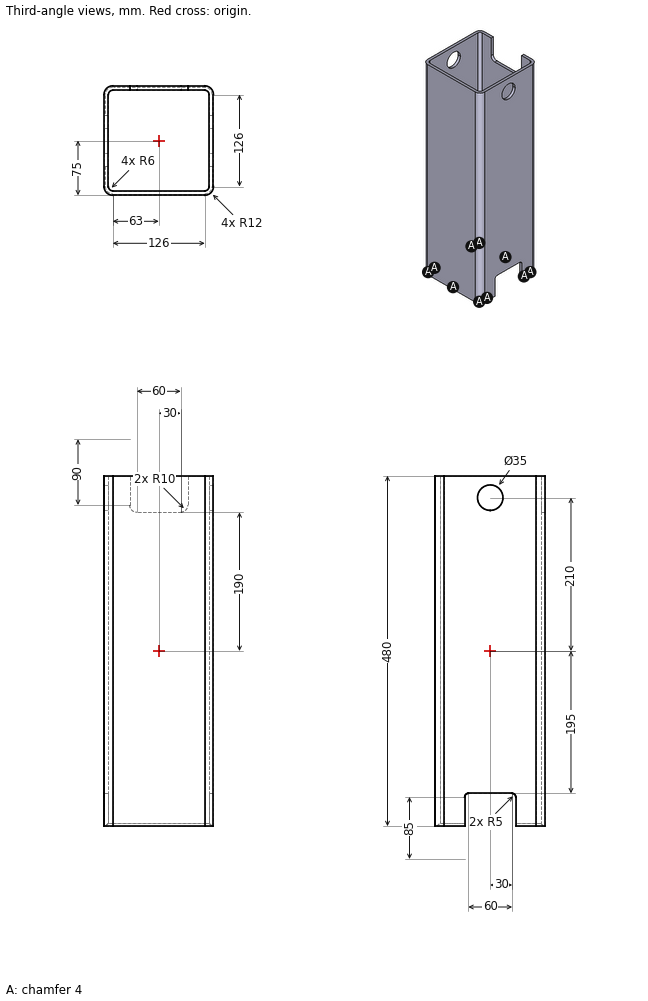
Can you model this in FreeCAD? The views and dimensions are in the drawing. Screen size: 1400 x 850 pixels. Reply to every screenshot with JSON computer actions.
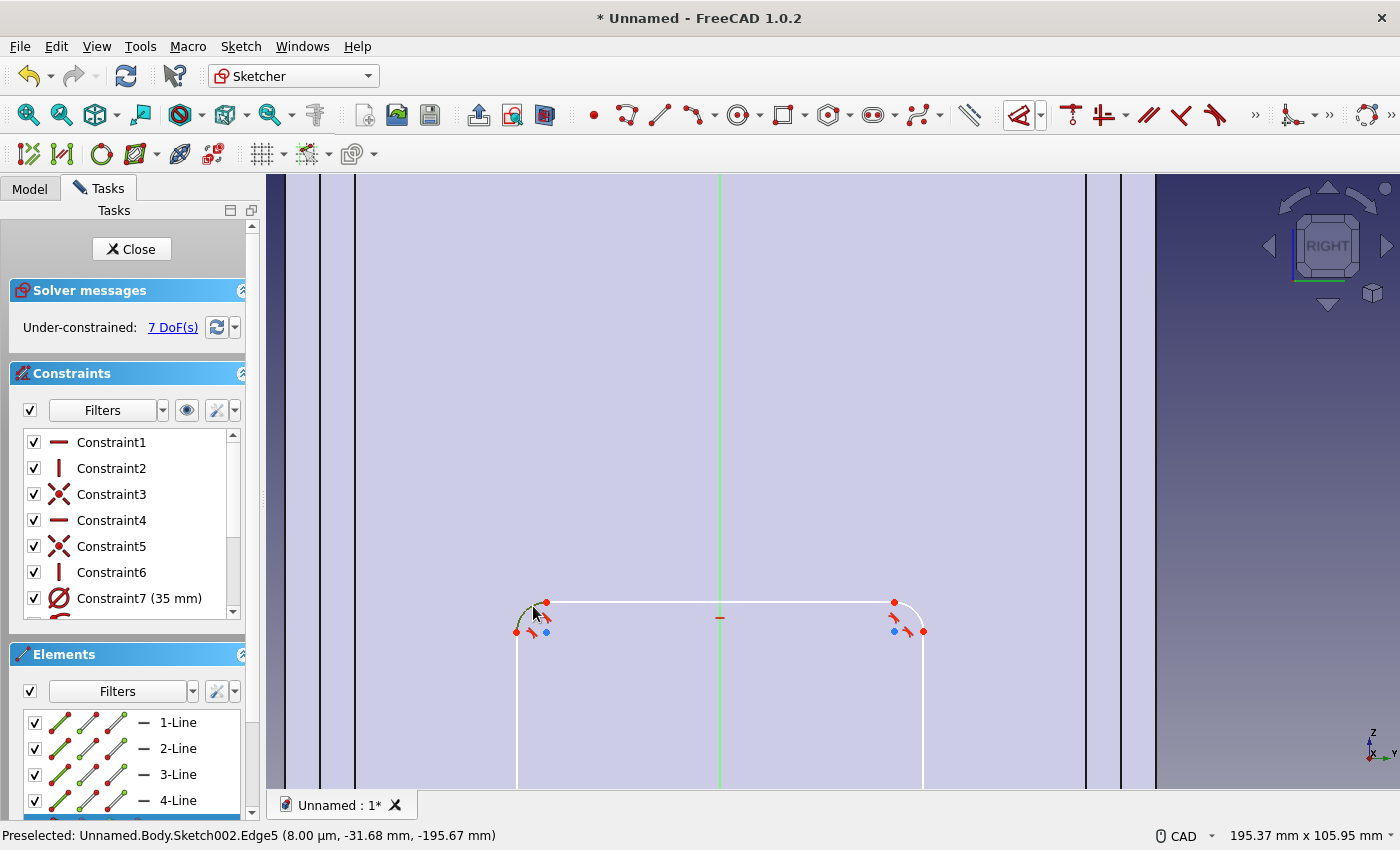
{"action": "left_click", "coordinate": [920, 619]}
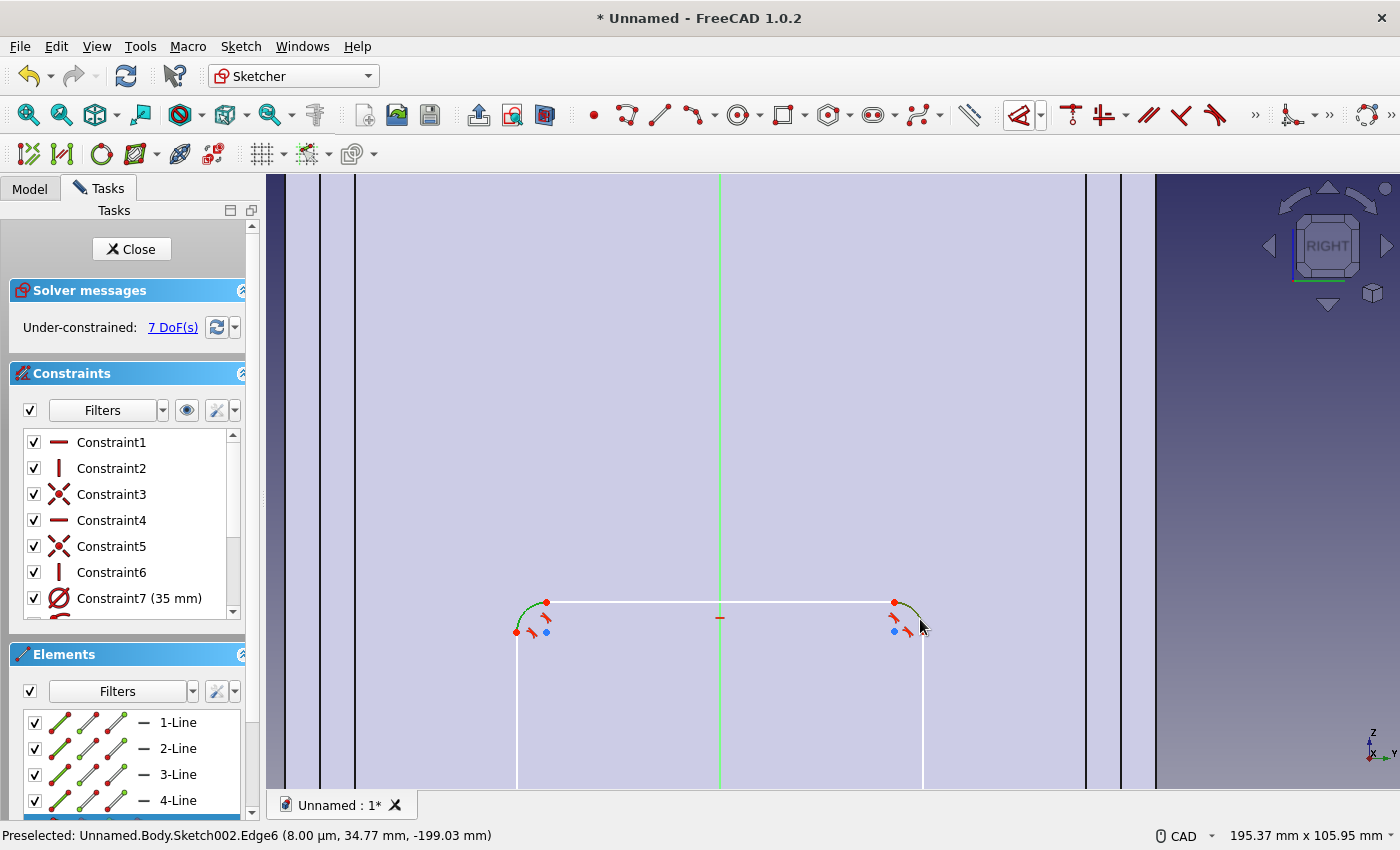
{"action": "key", "text": "e"}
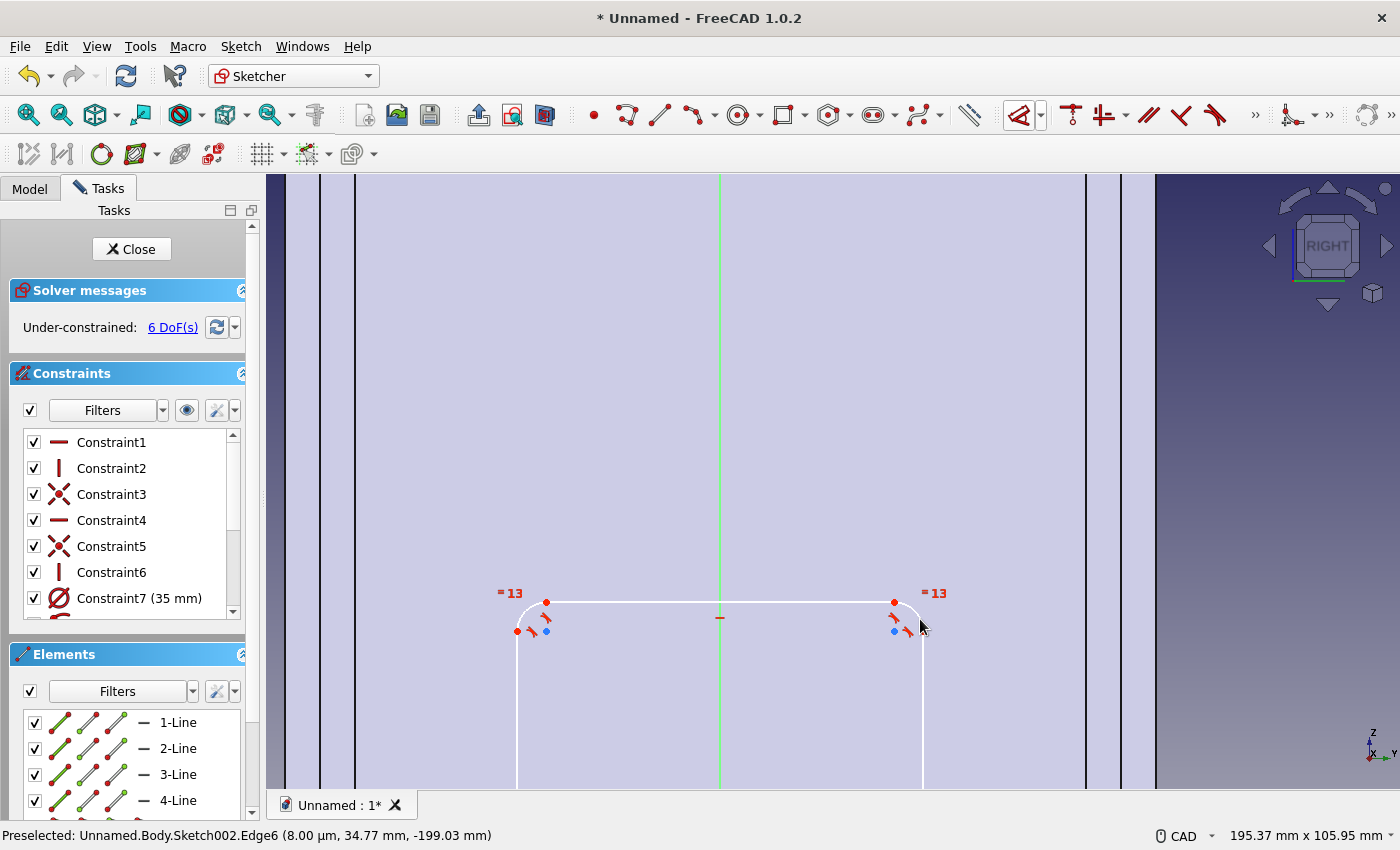
{"action": "scroll", "coordinate": [533, 606], "scroll_direction": "up", "scroll_amount": 2}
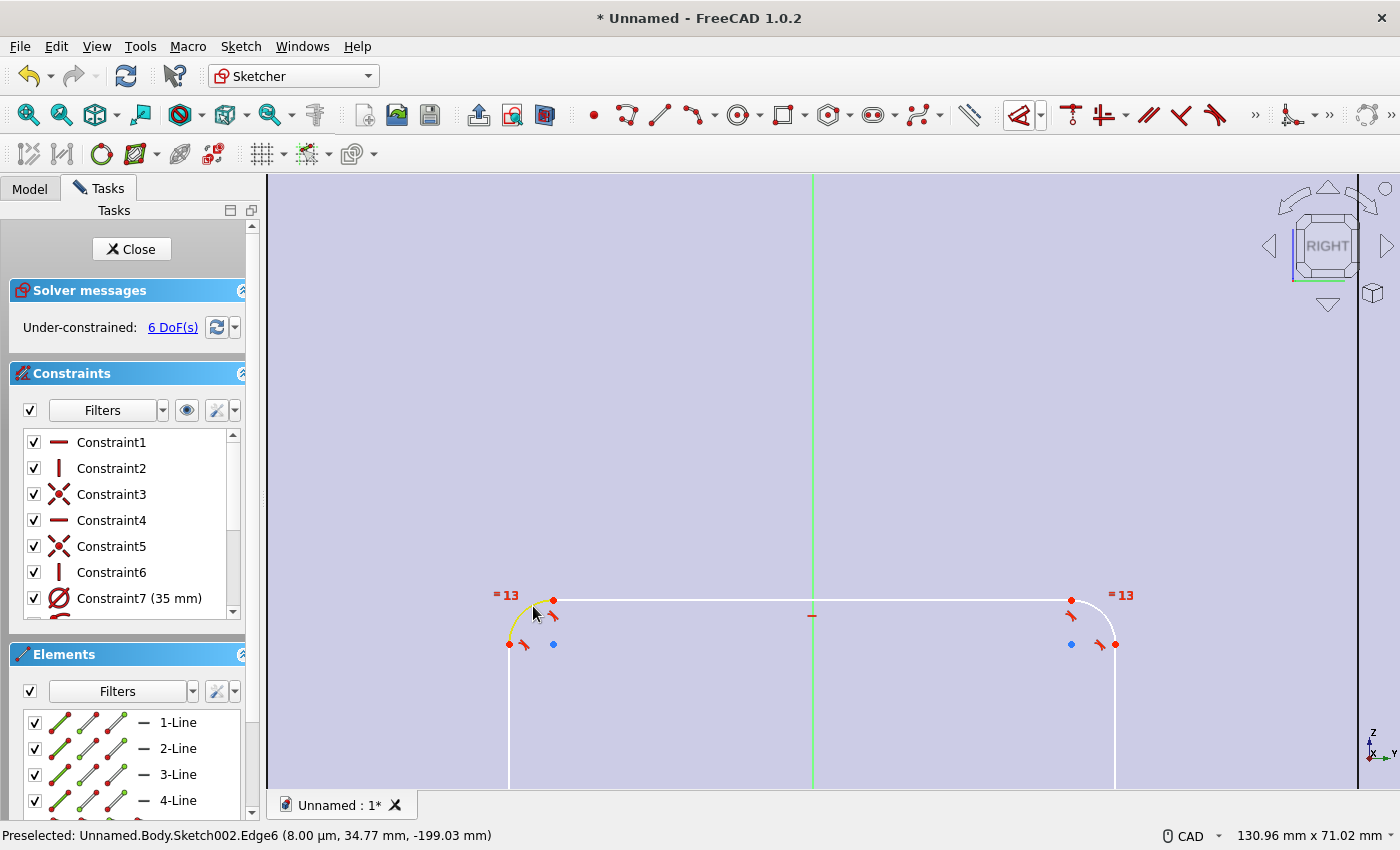
{"action": "left_click", "coordinate": [533, 605]}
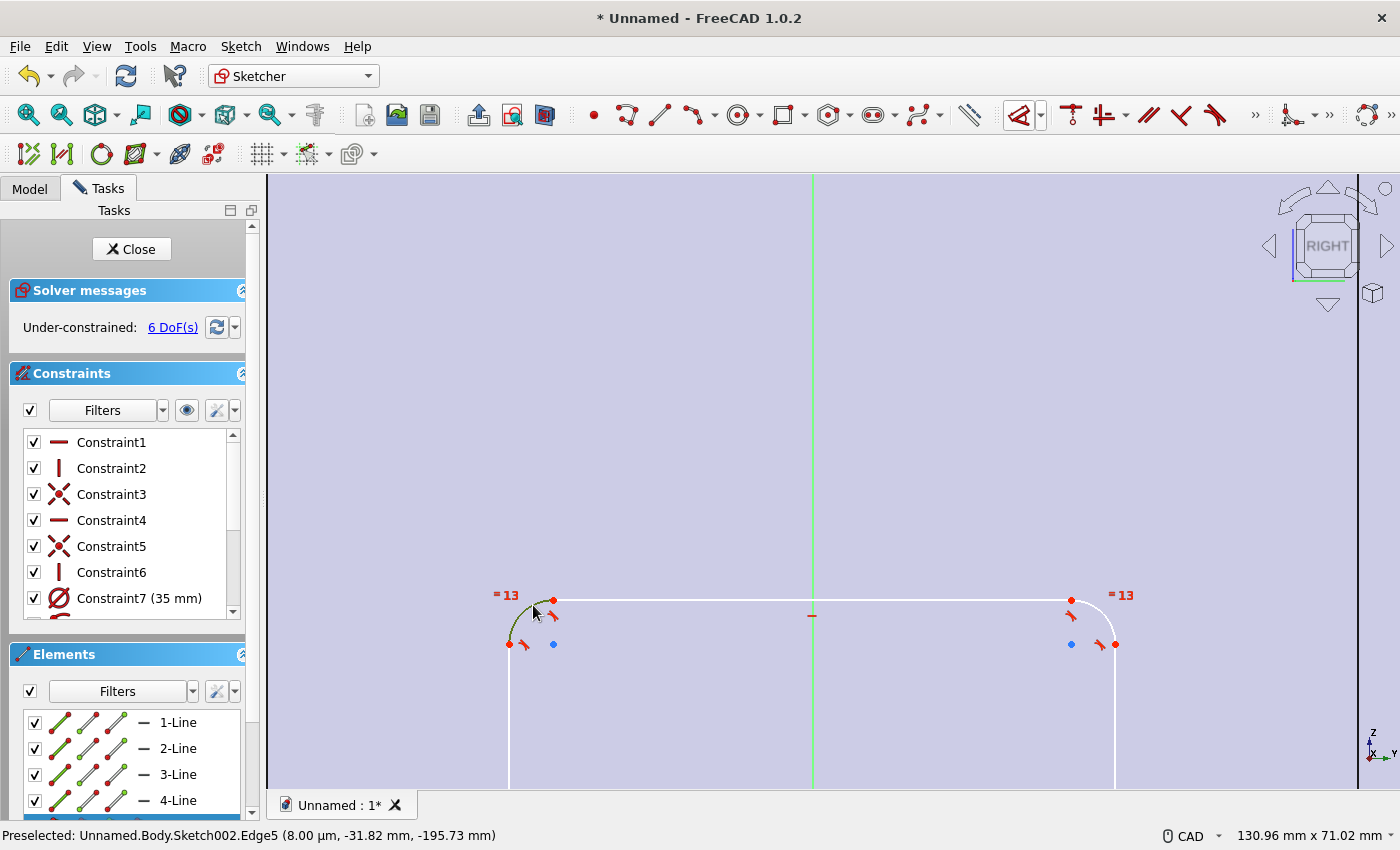
{"action": "left_click", "coordinate": [1040, 116]}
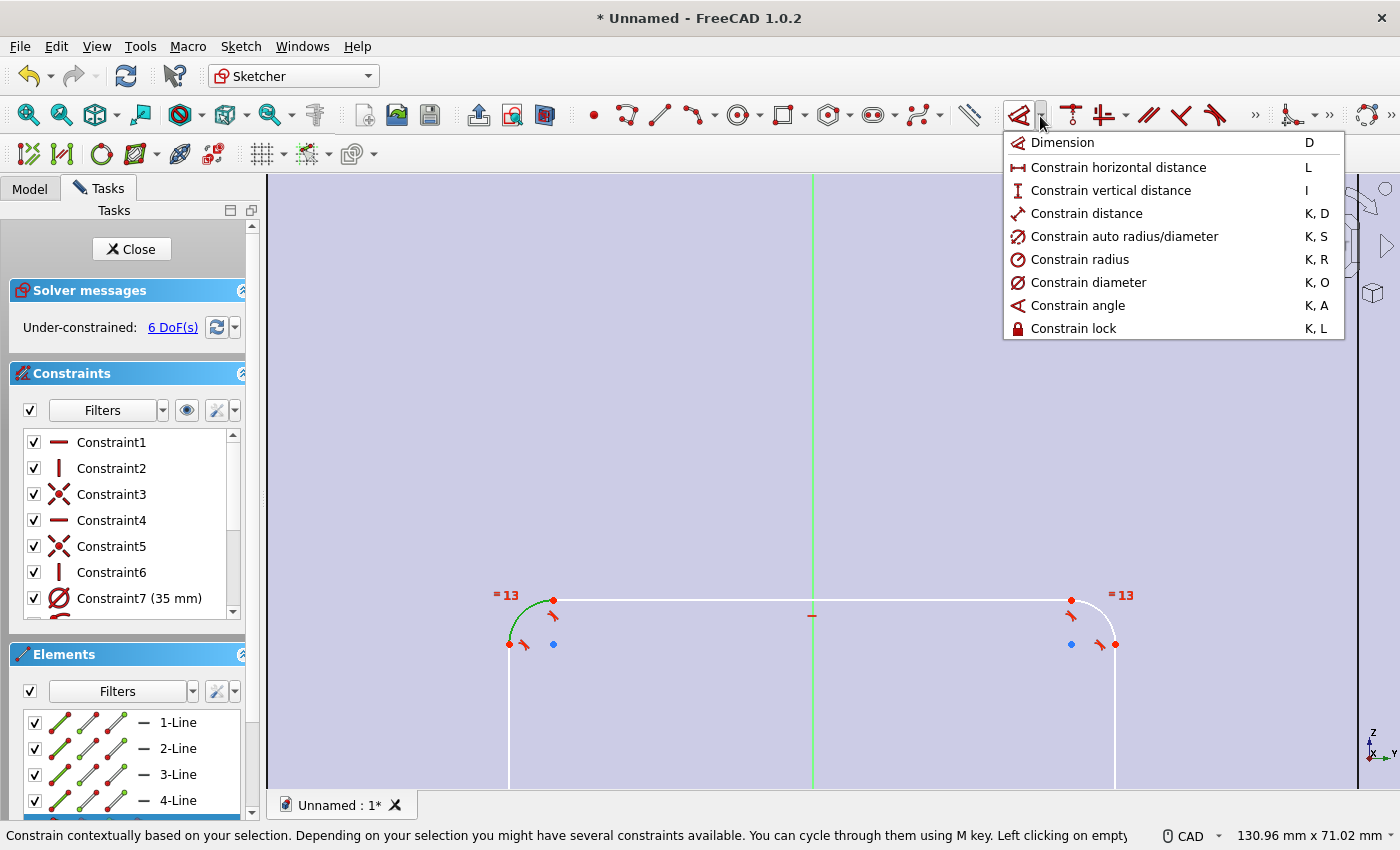
{"action": "left_click", "coordinate": [1174, 260]}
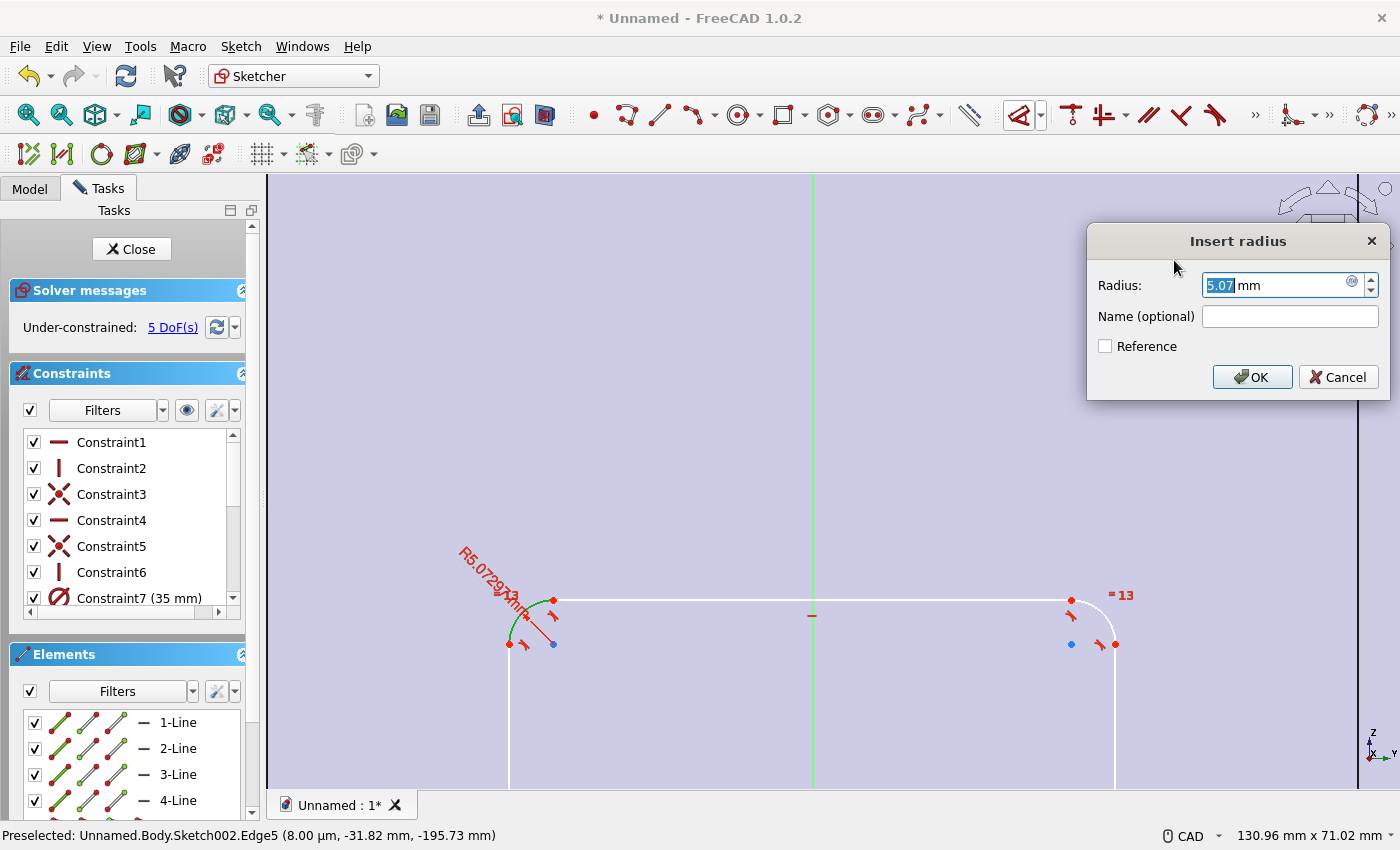
{"action": "type", "text": "5"}
{"action": "key", "text": "Return"}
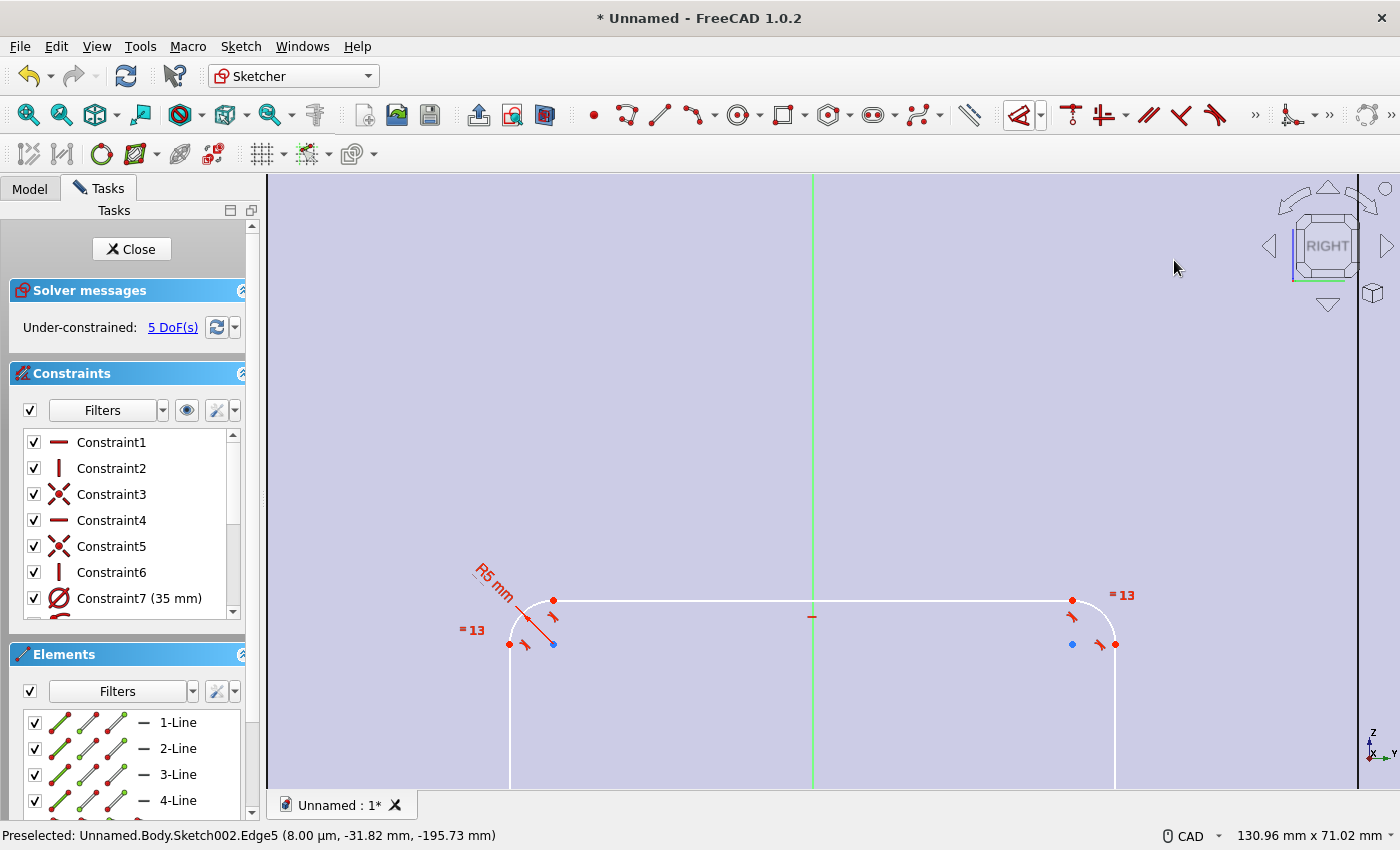
{"action": "scroll", "coordinate": [760, 614], "scroll_direction": "down", "scroll_amount": 12}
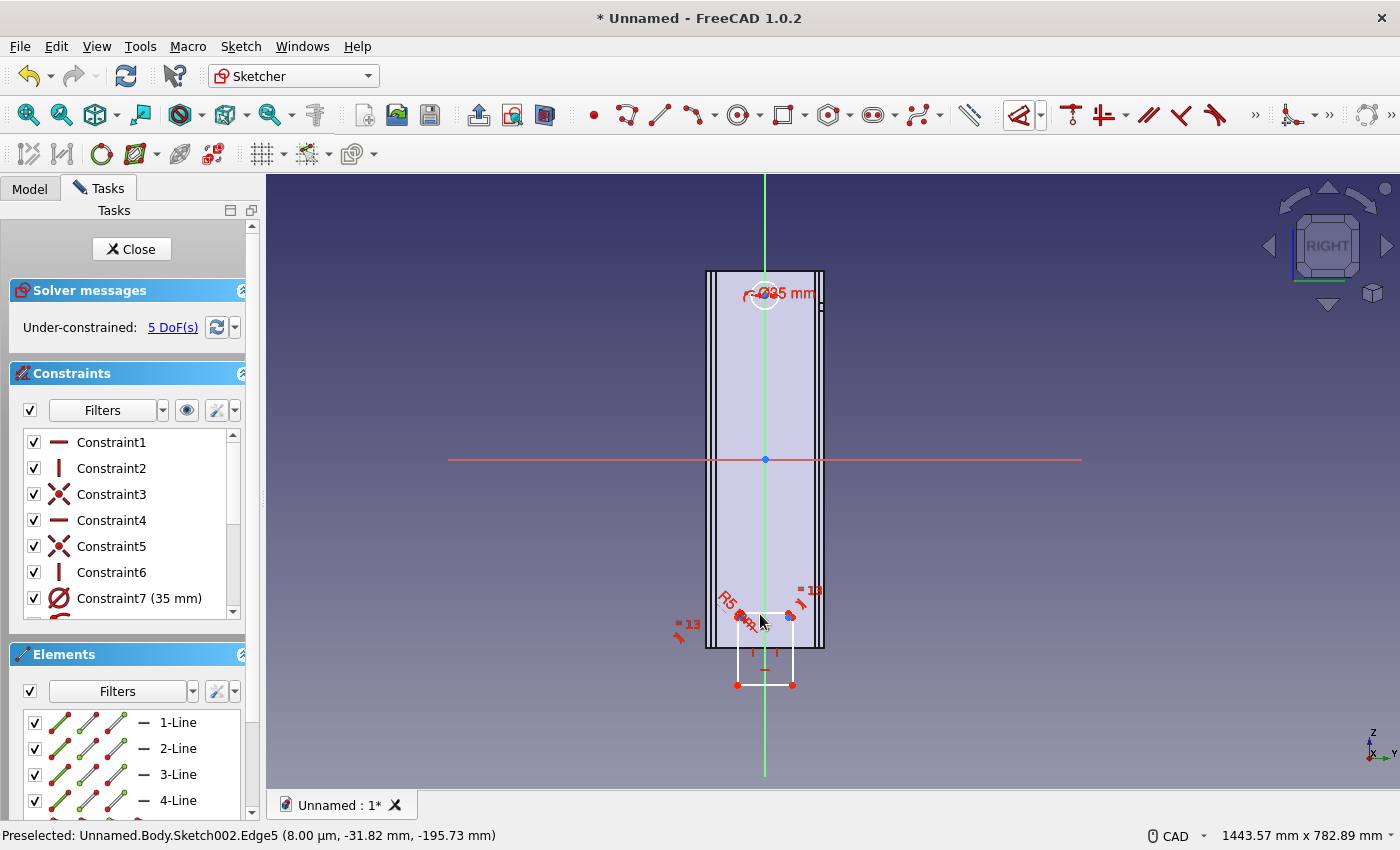
{"action": "scroll", "coordinate": [775, 613], "scroll_direction": "up", "scroll_amount": 2}